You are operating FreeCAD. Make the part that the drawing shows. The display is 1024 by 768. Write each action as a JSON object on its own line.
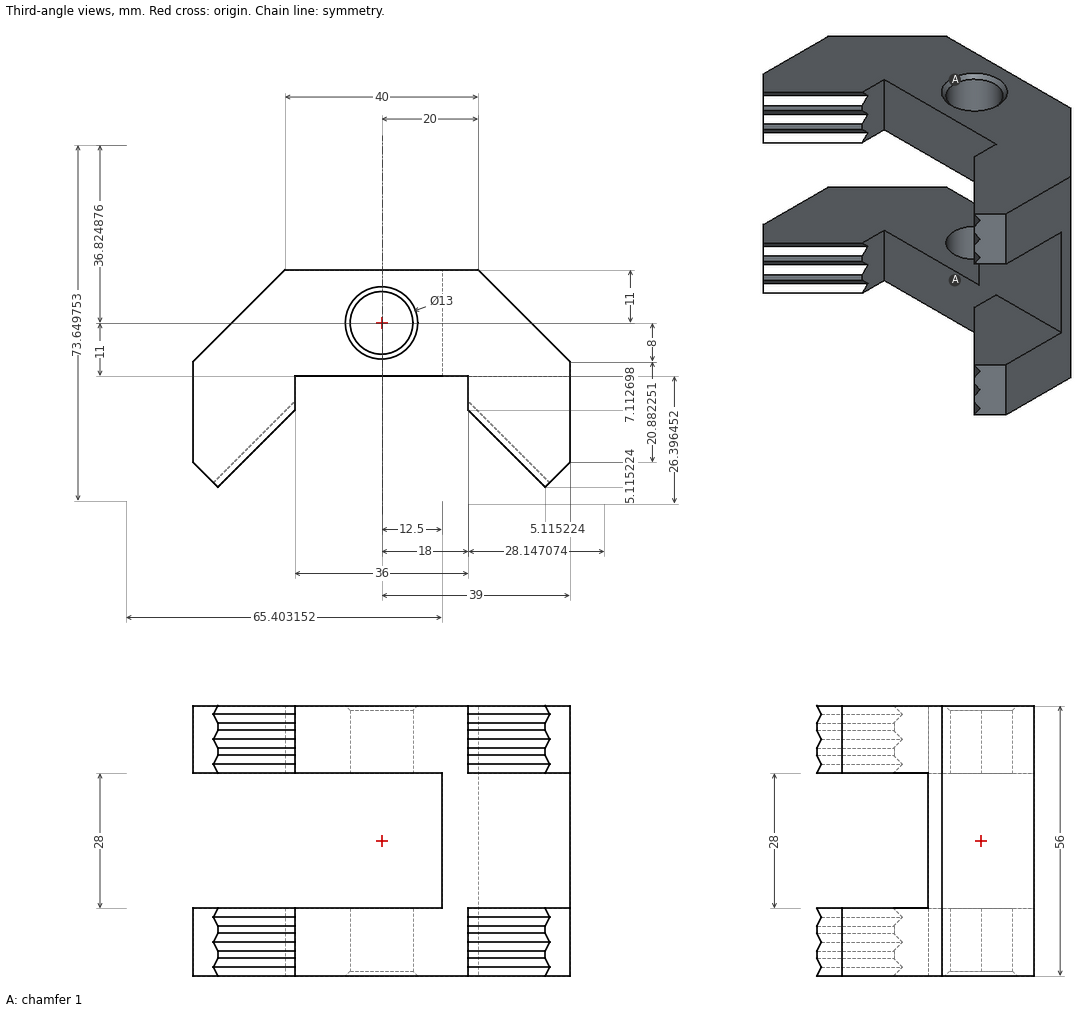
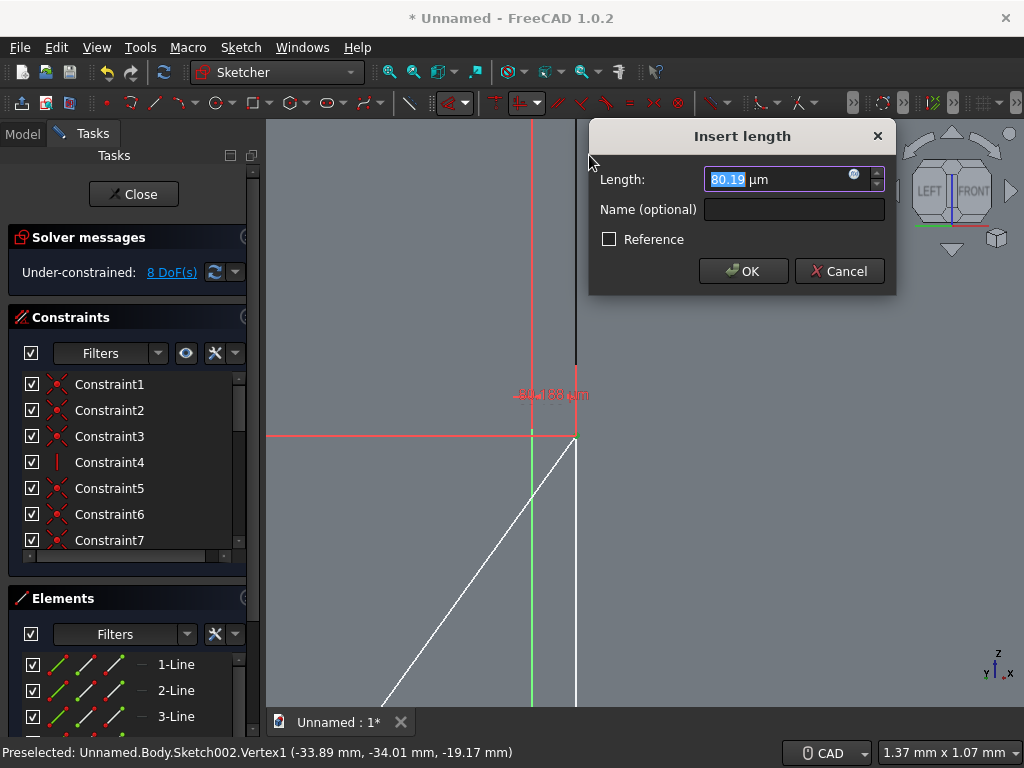
{"action": "key", "text": "ctrl+a"}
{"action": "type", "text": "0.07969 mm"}
{"action": "key", "text": "Return"}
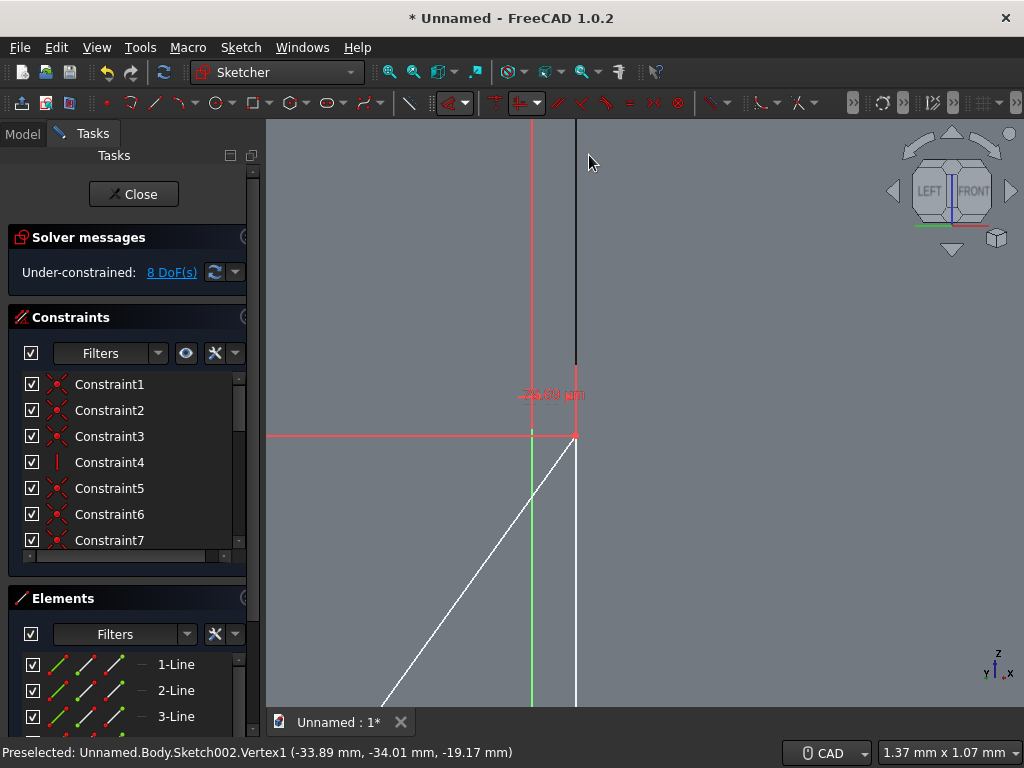
{"action": "scroll", "coordinate": [587, 492], "scroll_direction": "down", "scroll_amount": 18}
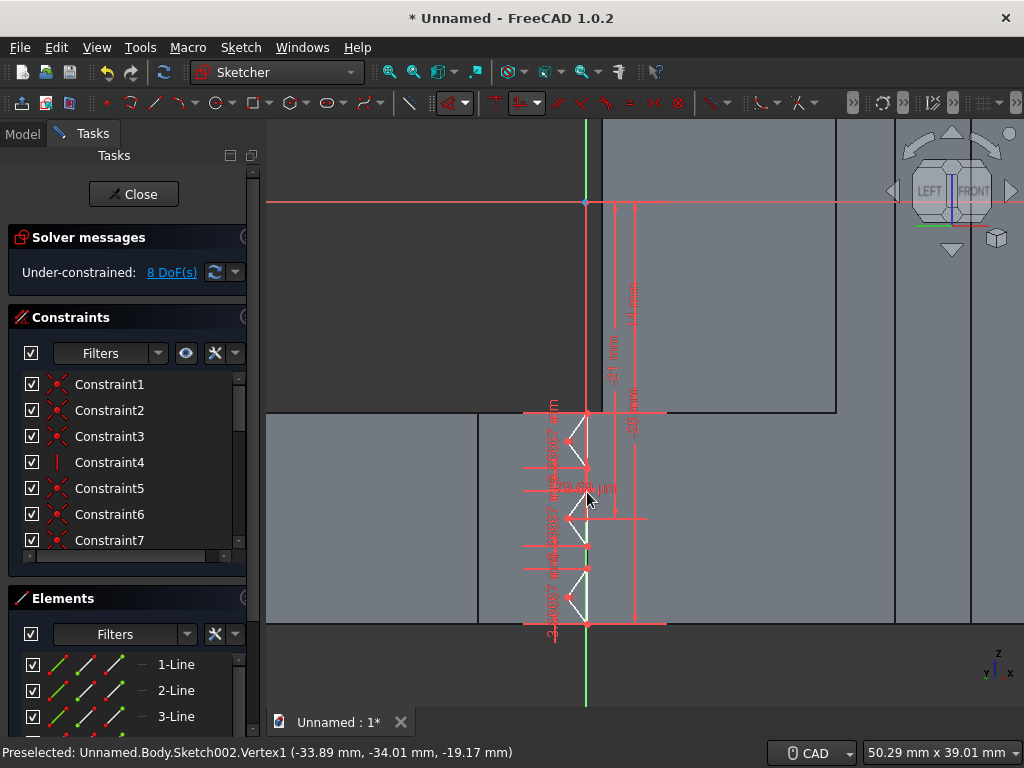
{"action": "scroll", "coordinate": [587, 413], "scroll_direction": "up", "scroll_amount": 18}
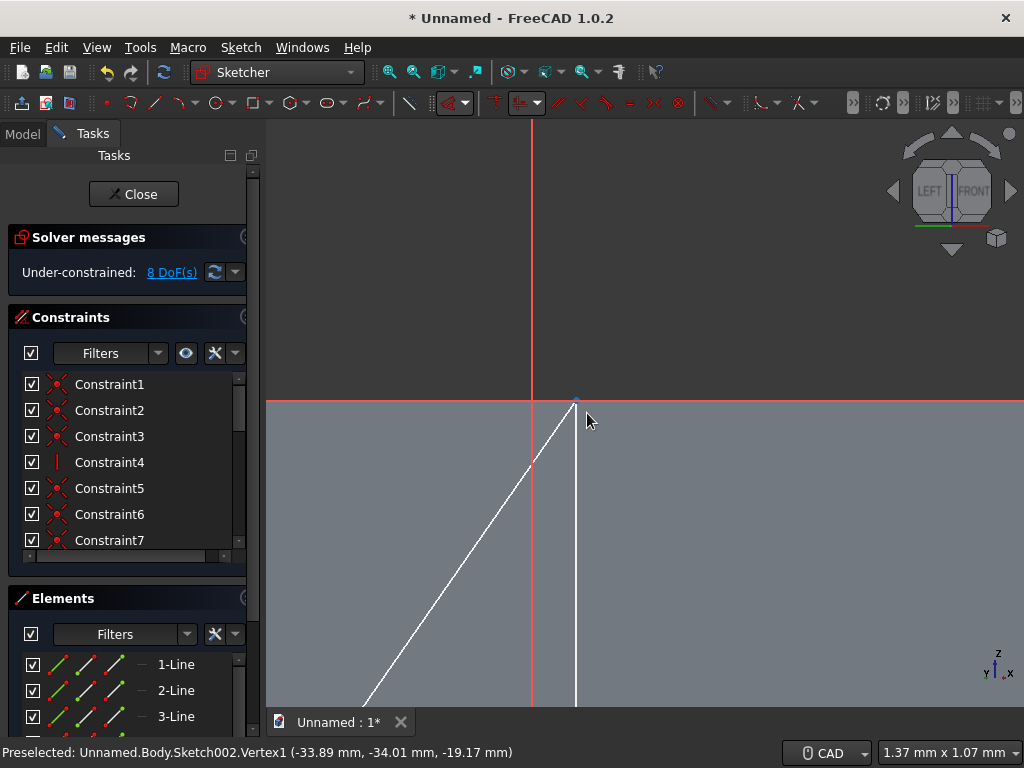
{"action": "left_click", "coordinate": [576, 401]}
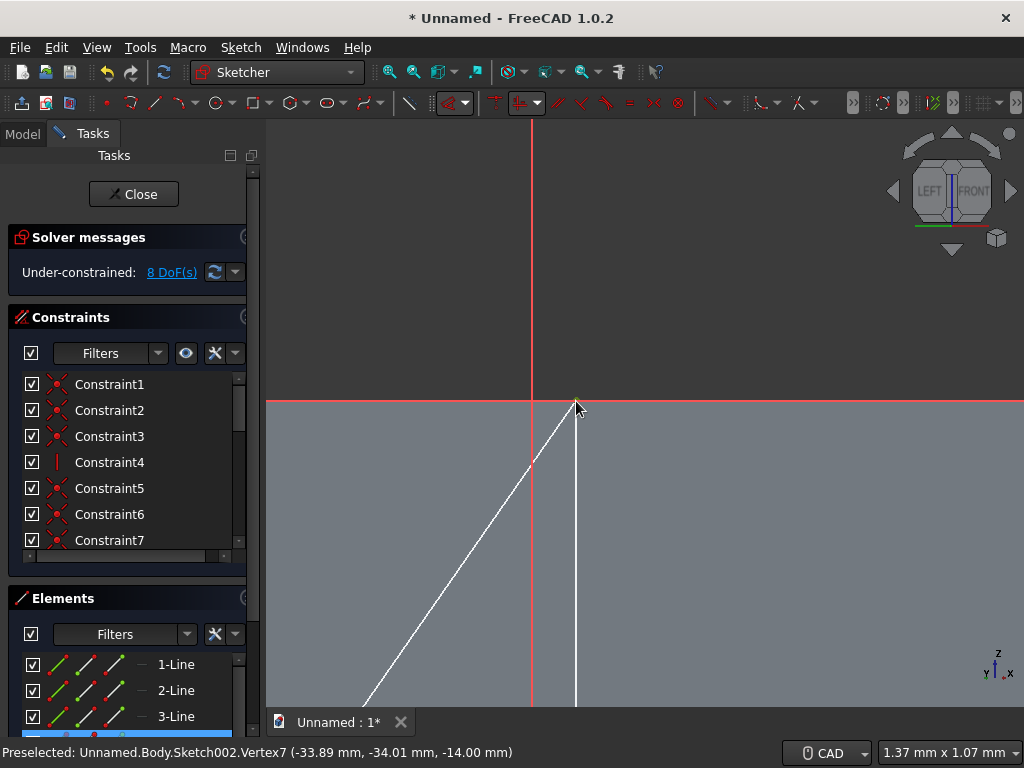
{"action": "key", "text": "l"}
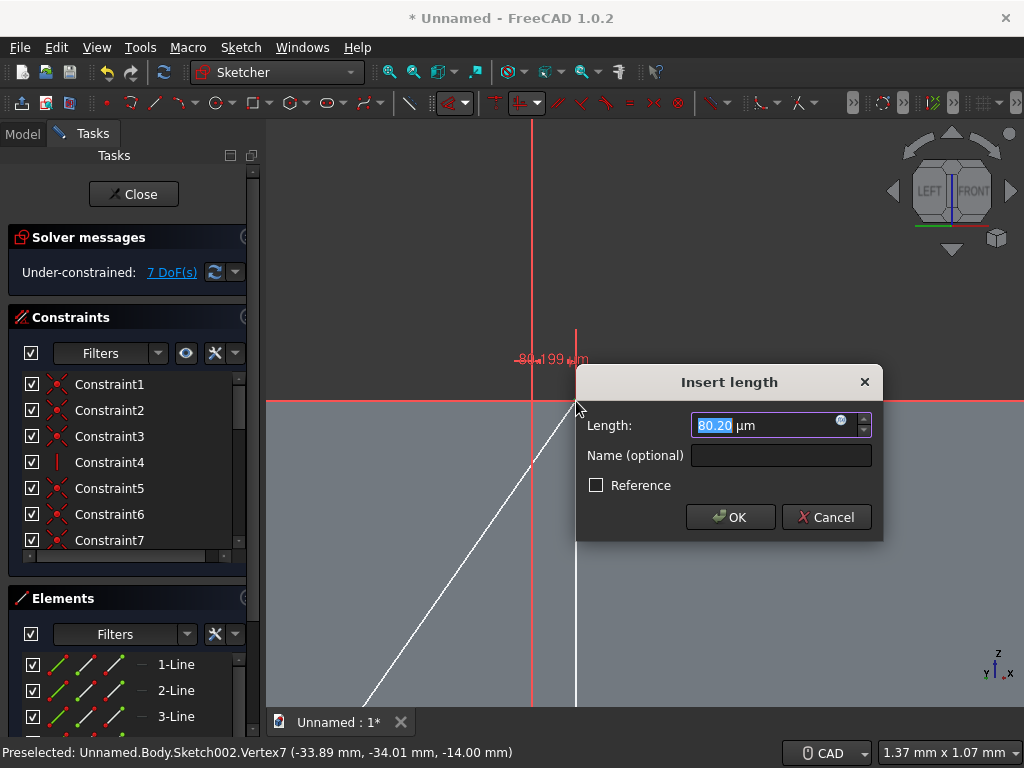
{"action": "key", "text": "ctrl+a"}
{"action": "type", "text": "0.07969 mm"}
{"action": "key", "text": "Return"}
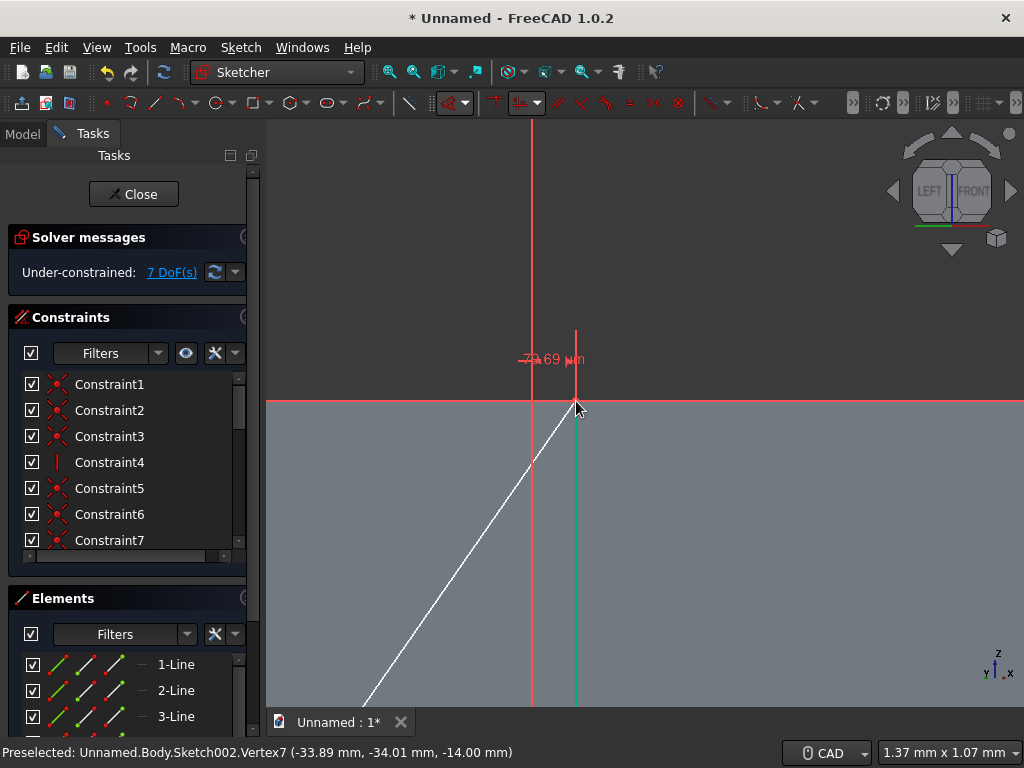
{"action": "scroll", "coordinate": [587, 413], "scroll_direction": "down", "scroll_amount": 18}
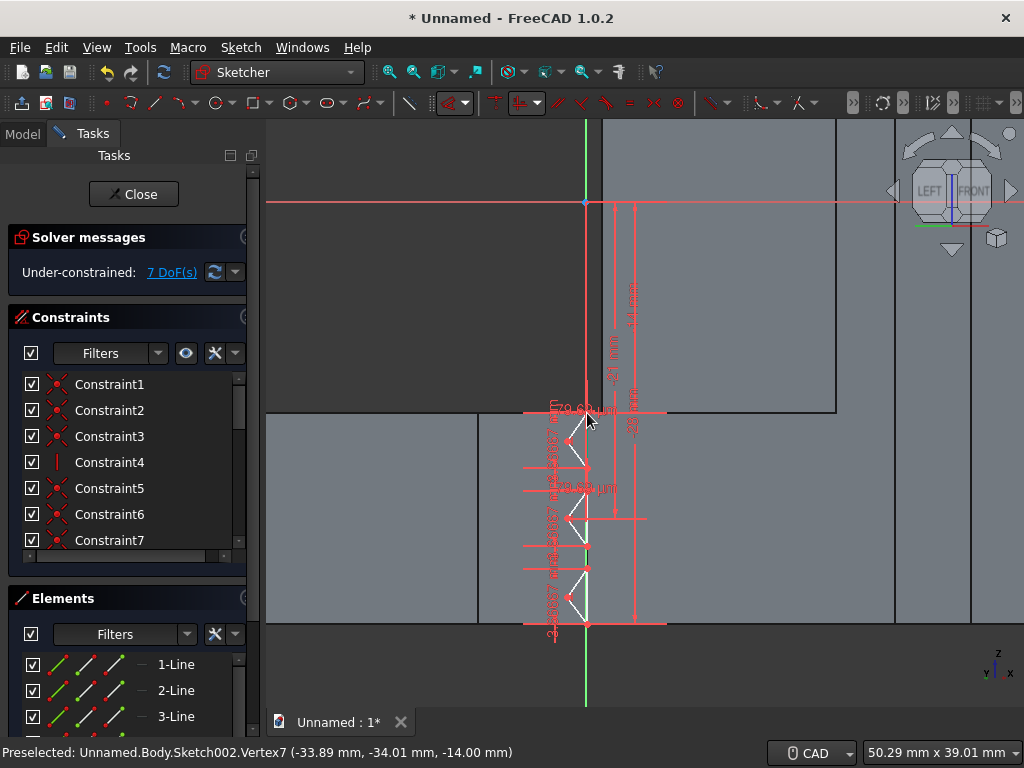
{"action": "scroll", "coordinate": [587, 569], "scroll_direction": "up", "scroll_amount": 18}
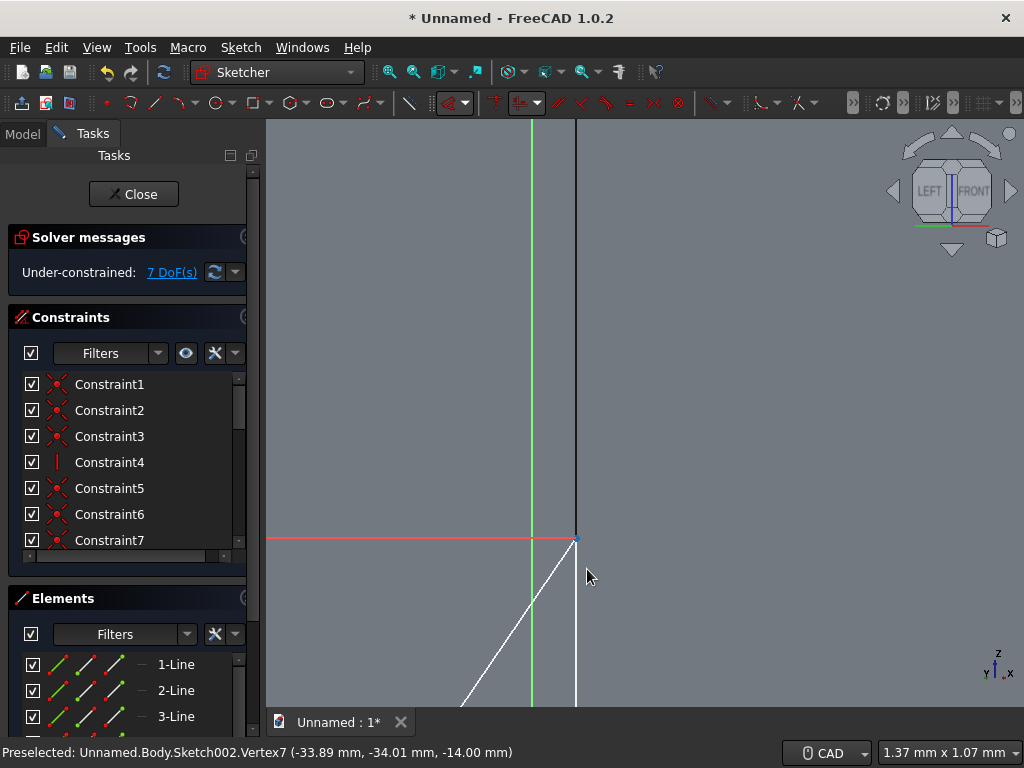
{"action": "left_click", "coordinate": [576, 538]}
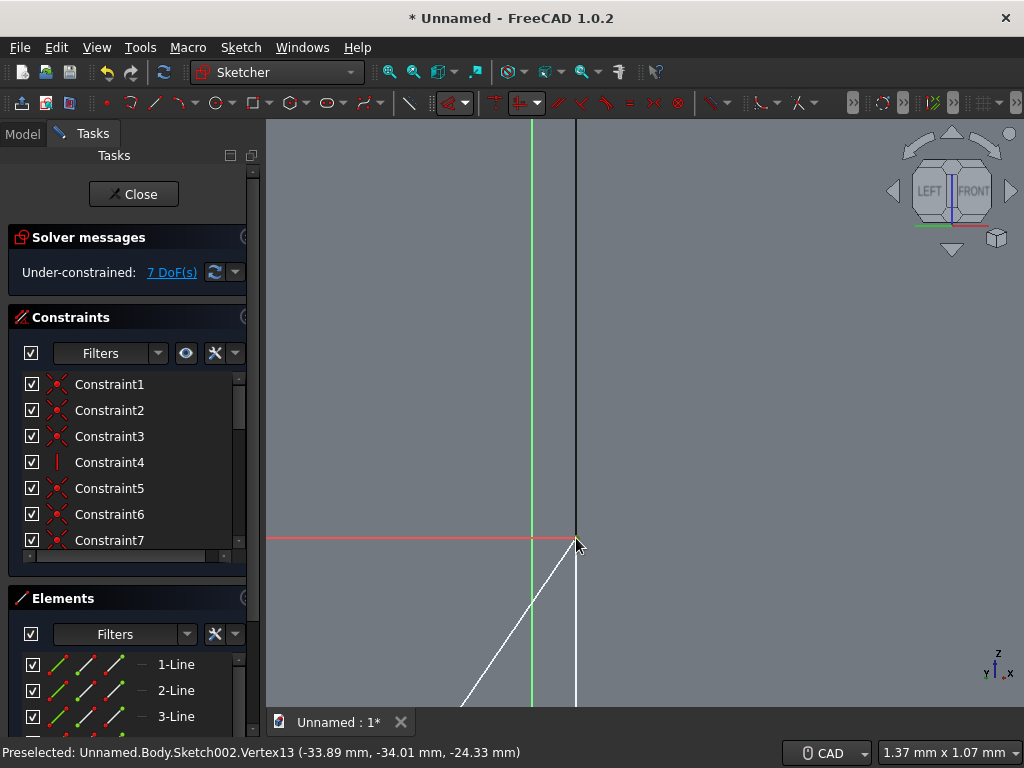
{"action": "left_click", "coordinate": [468, 104]}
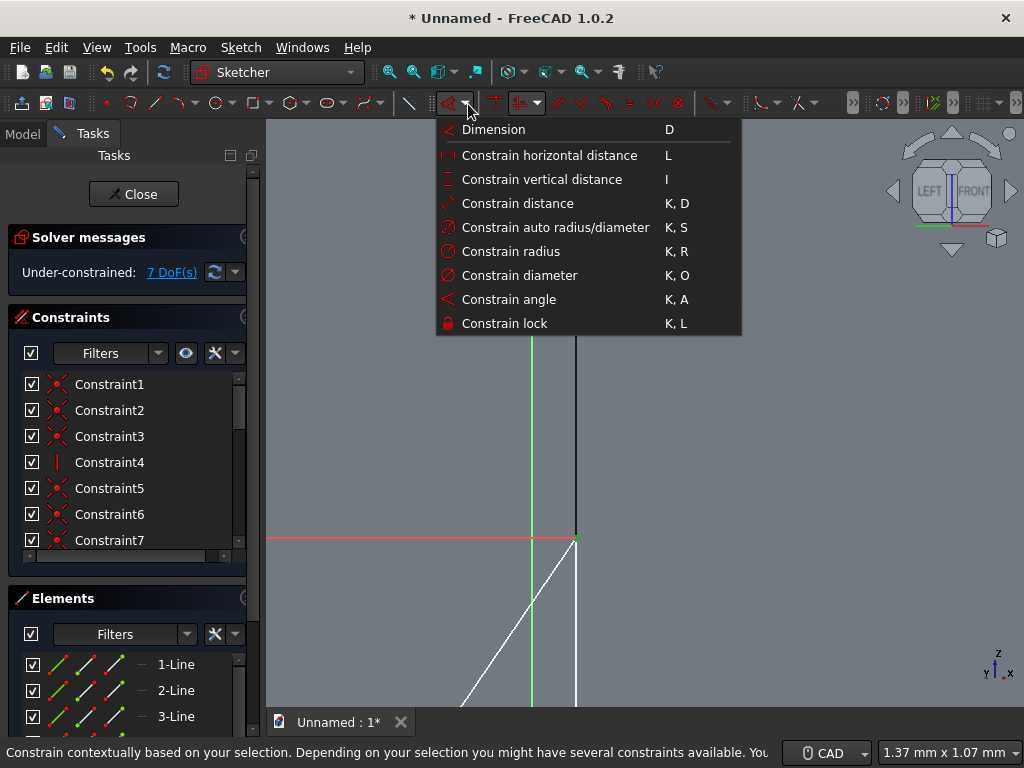
{"action": "left_click", "coordinate": [589, 155]}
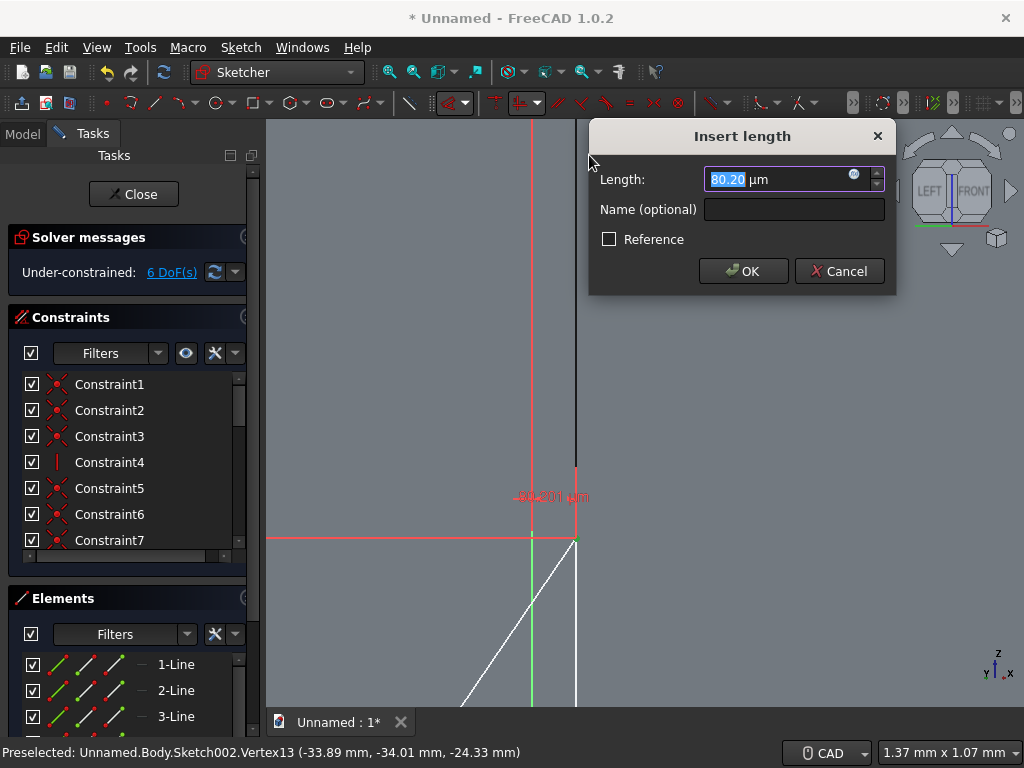
{"action": "key", "text": "ctrl+a"}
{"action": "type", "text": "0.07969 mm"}
{"action": "key", "text": "Return"}